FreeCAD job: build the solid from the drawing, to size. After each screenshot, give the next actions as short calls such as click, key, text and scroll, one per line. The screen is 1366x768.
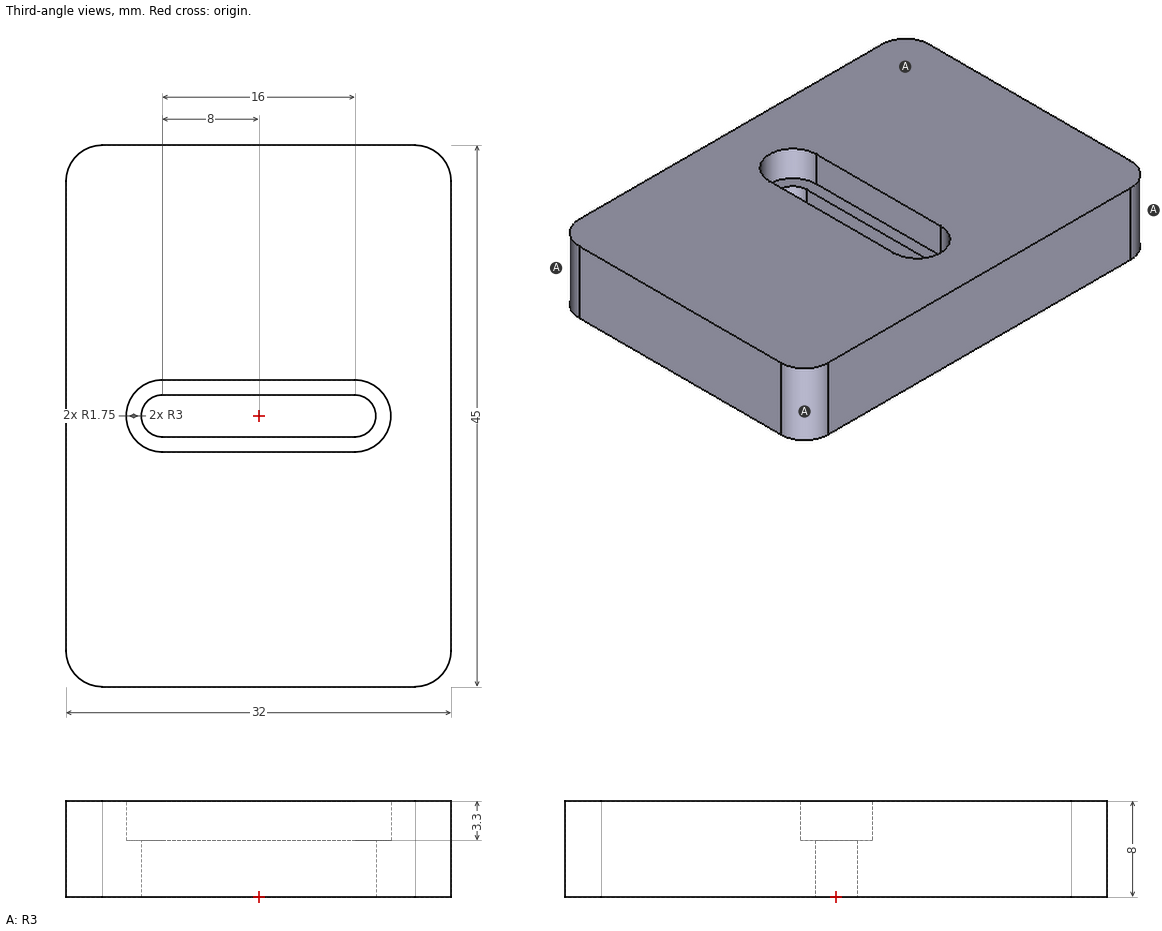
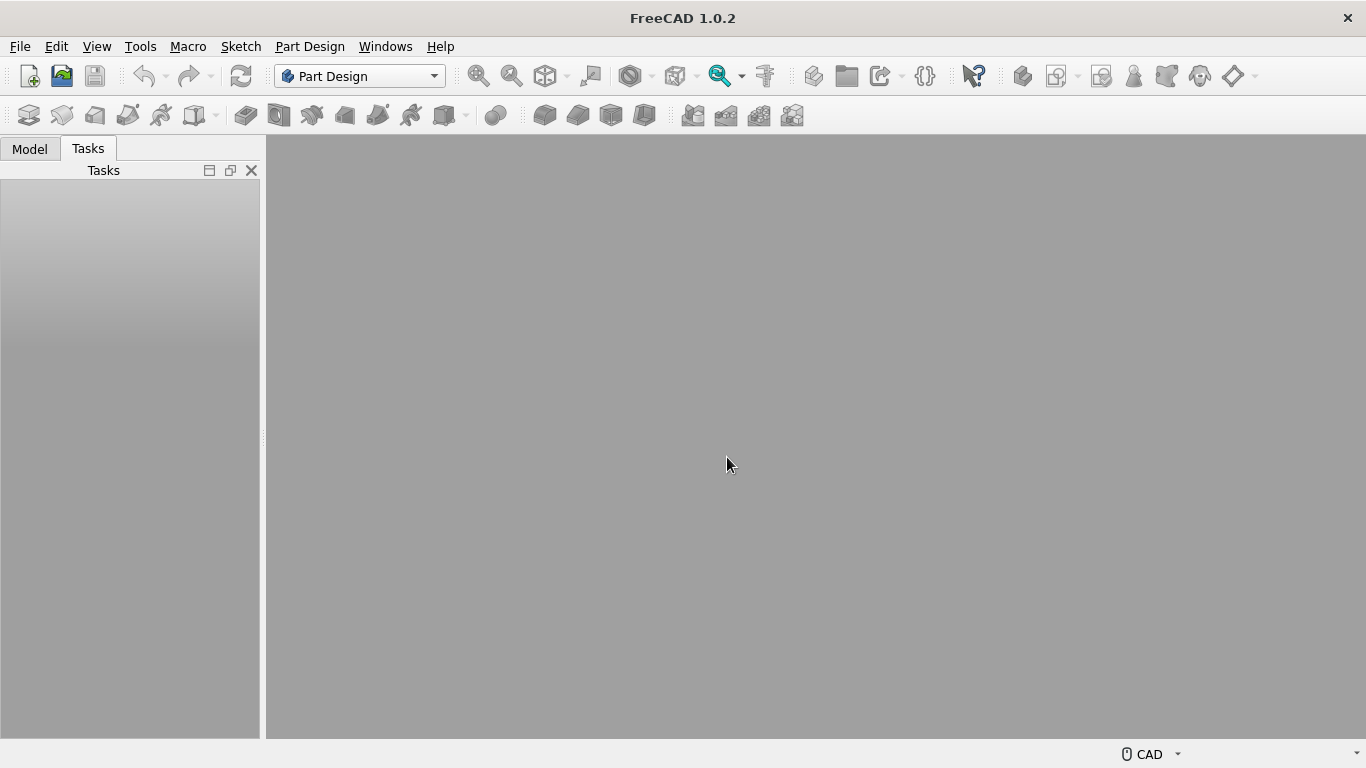
click(29, 76)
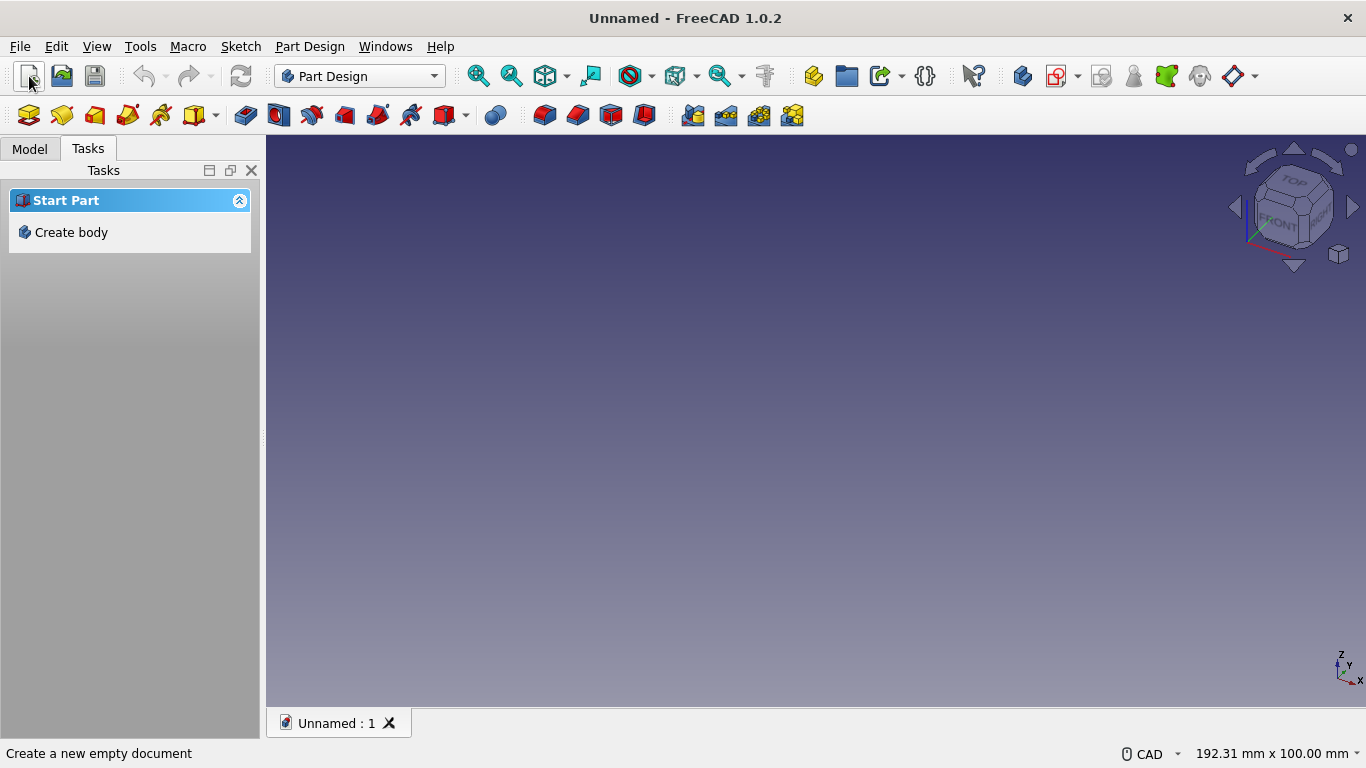
click(1056, 76)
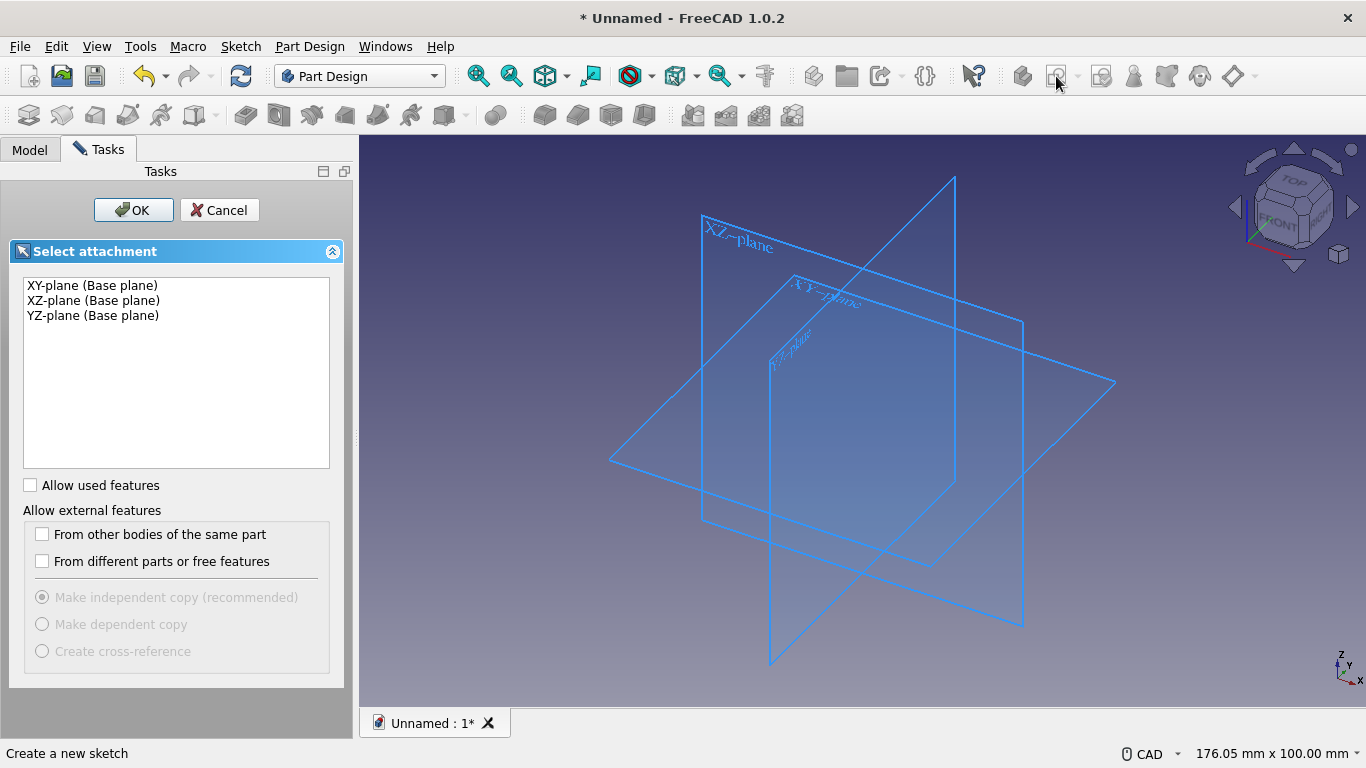
click(84, 286)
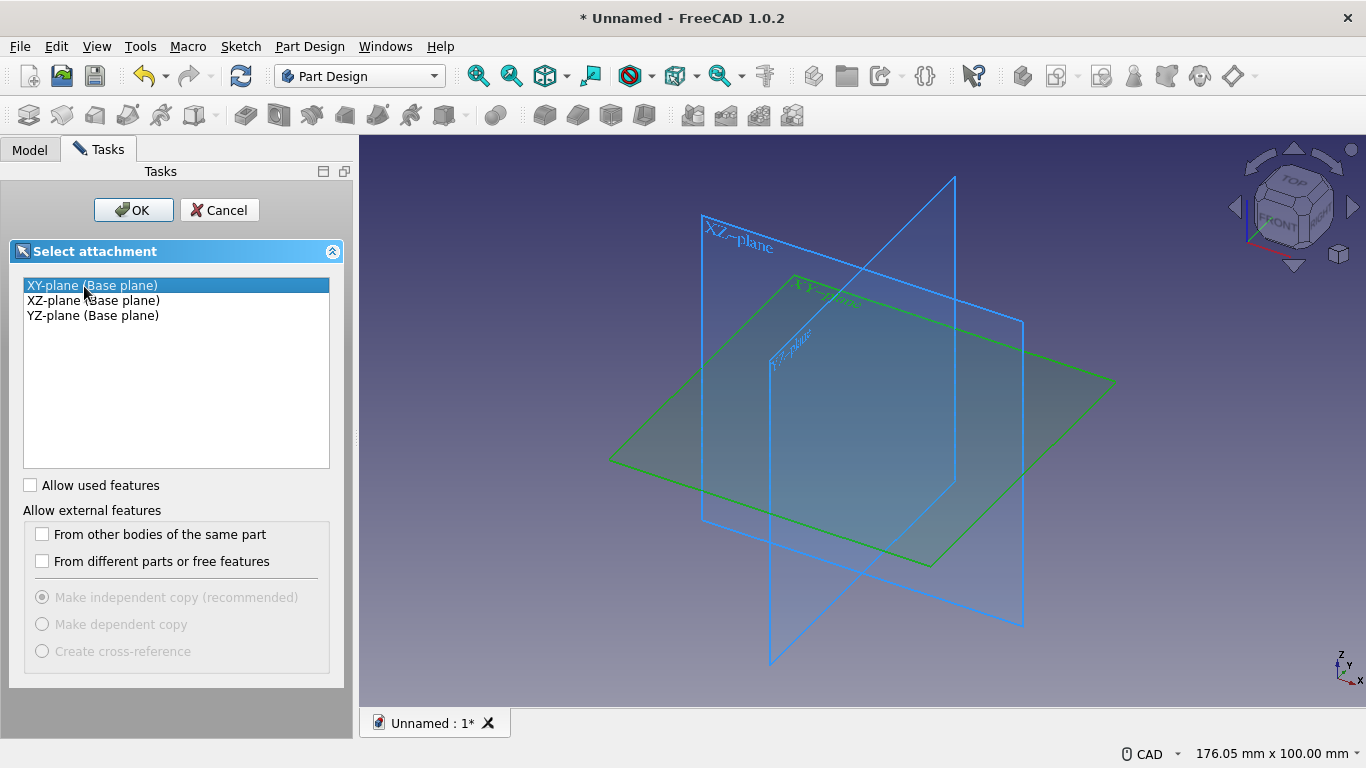
click(134, 210)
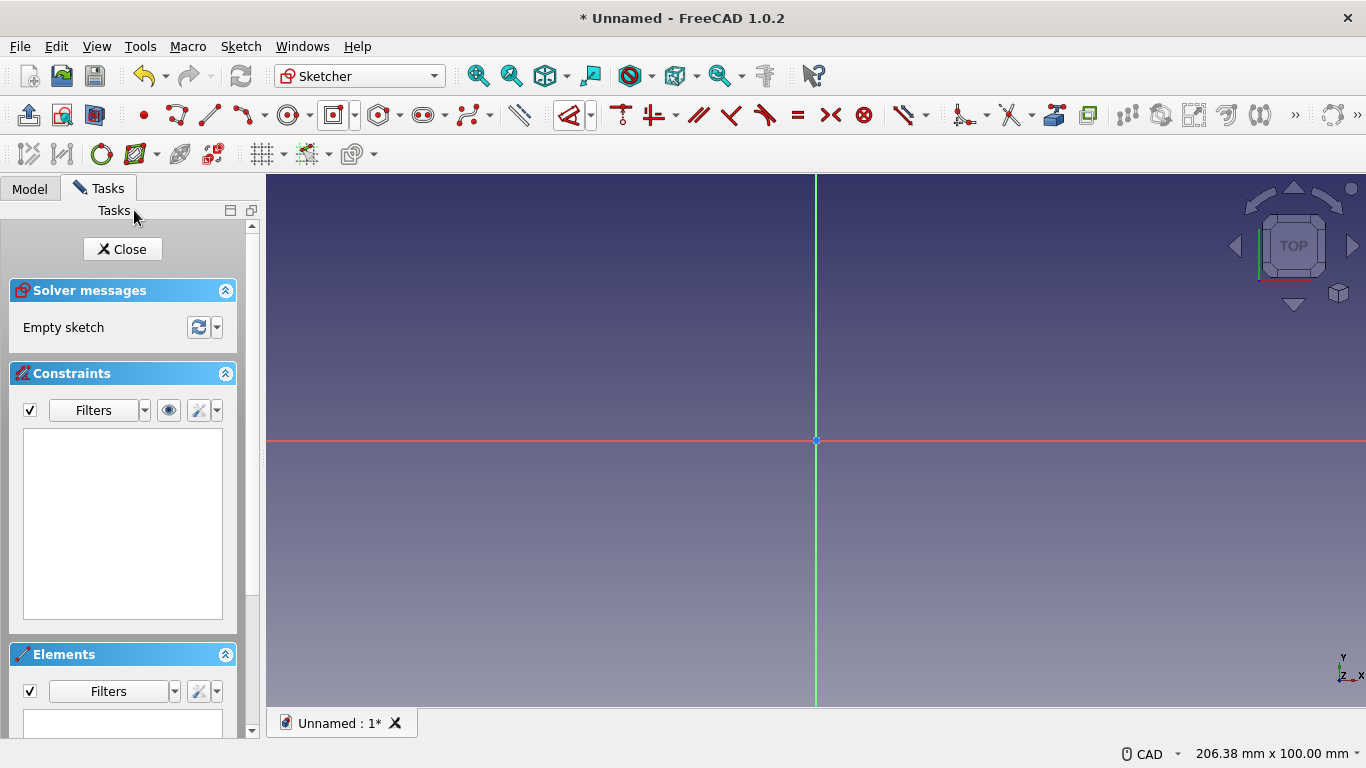
scroll(955, 440, up, 2)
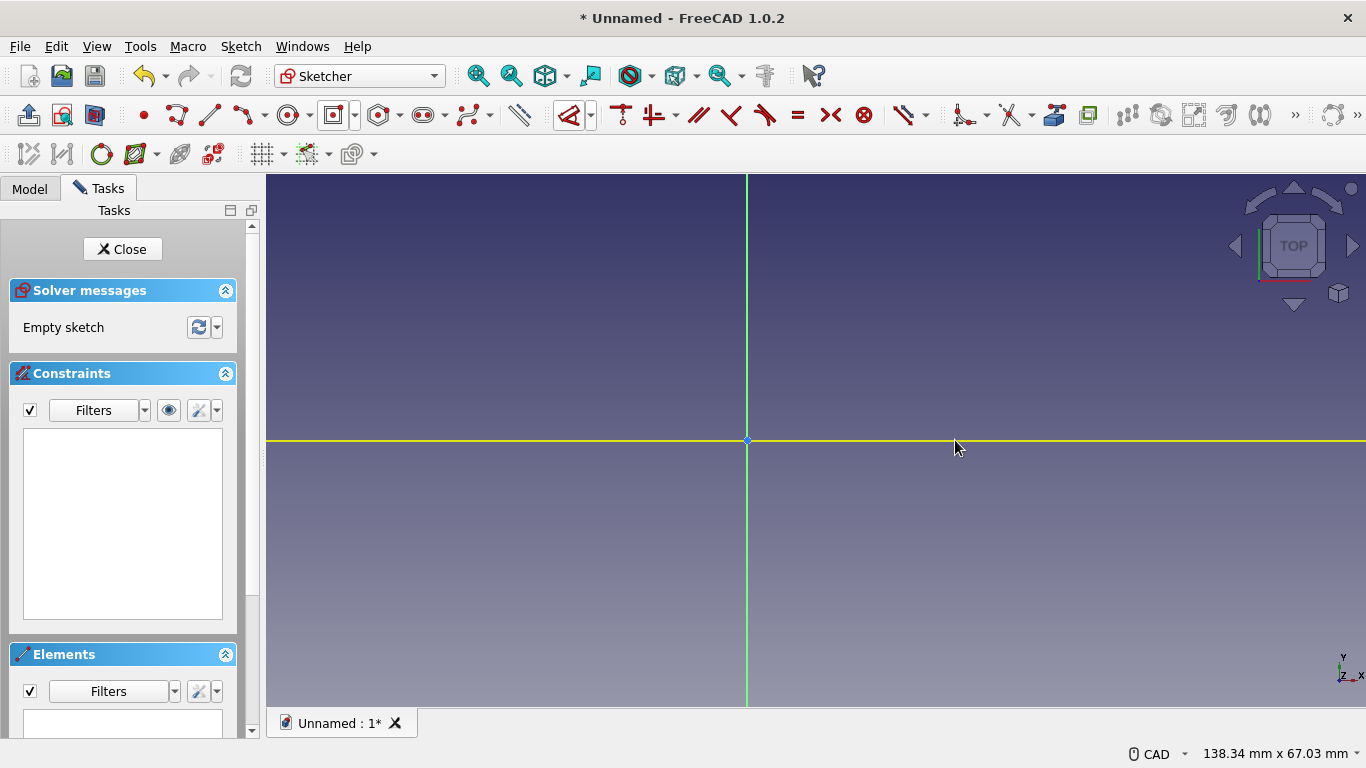
click(332, 116)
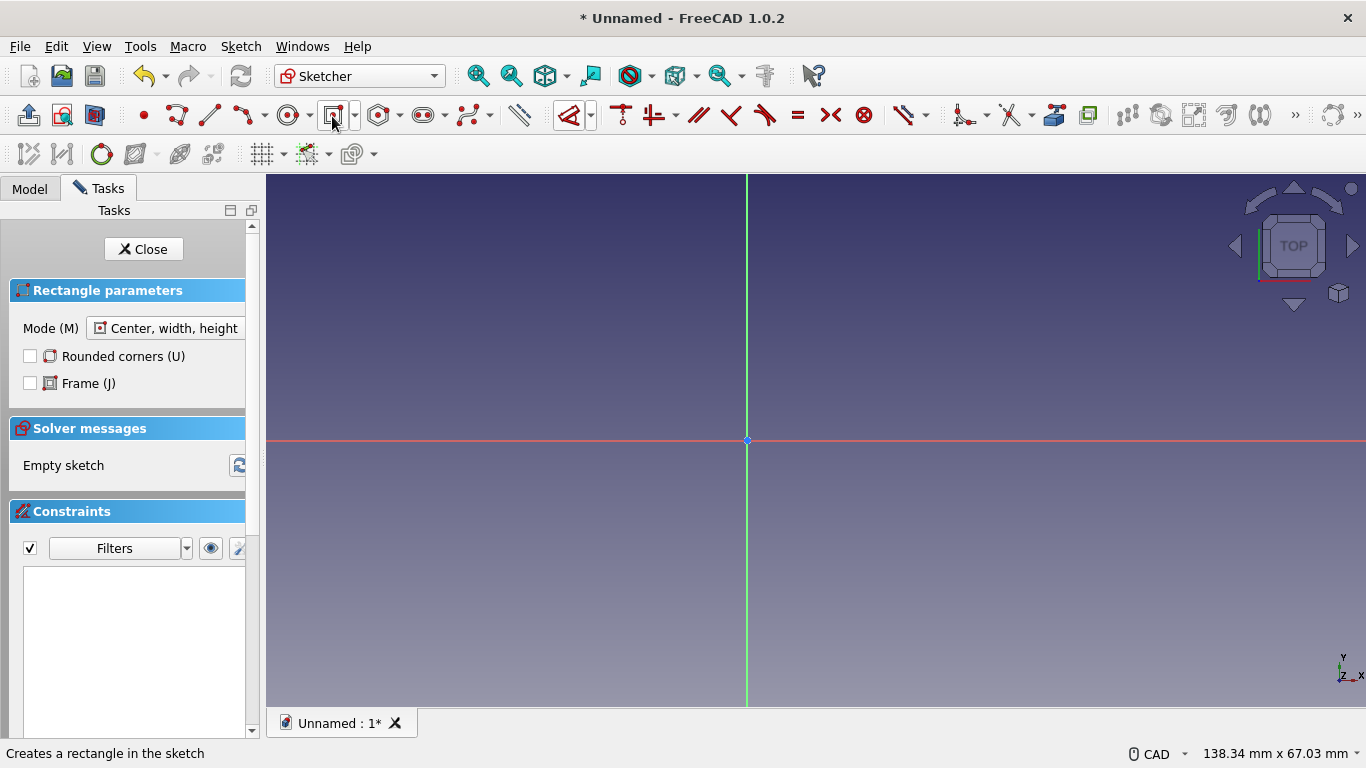
click(747, 440)
click(875, 262)
key(Escape)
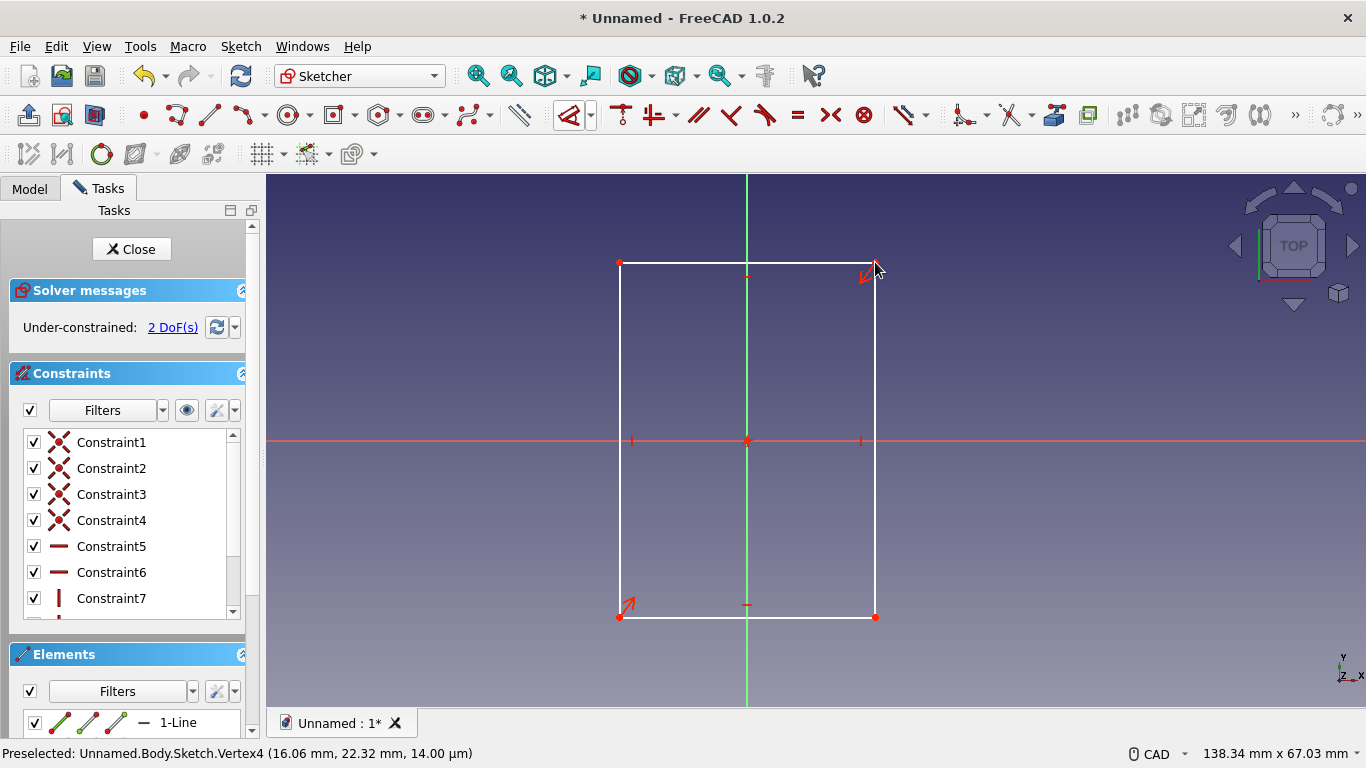
key(d)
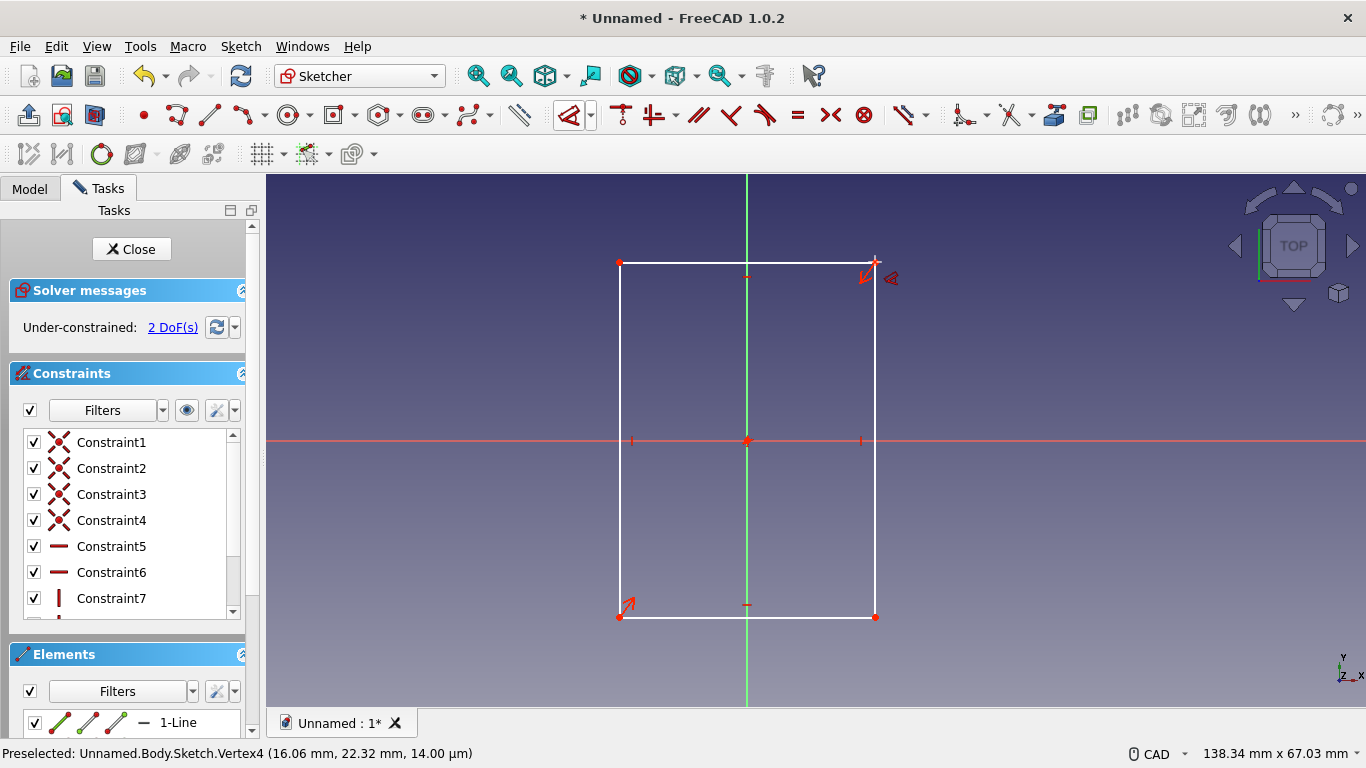
click(696, 618)
click(689, 652)